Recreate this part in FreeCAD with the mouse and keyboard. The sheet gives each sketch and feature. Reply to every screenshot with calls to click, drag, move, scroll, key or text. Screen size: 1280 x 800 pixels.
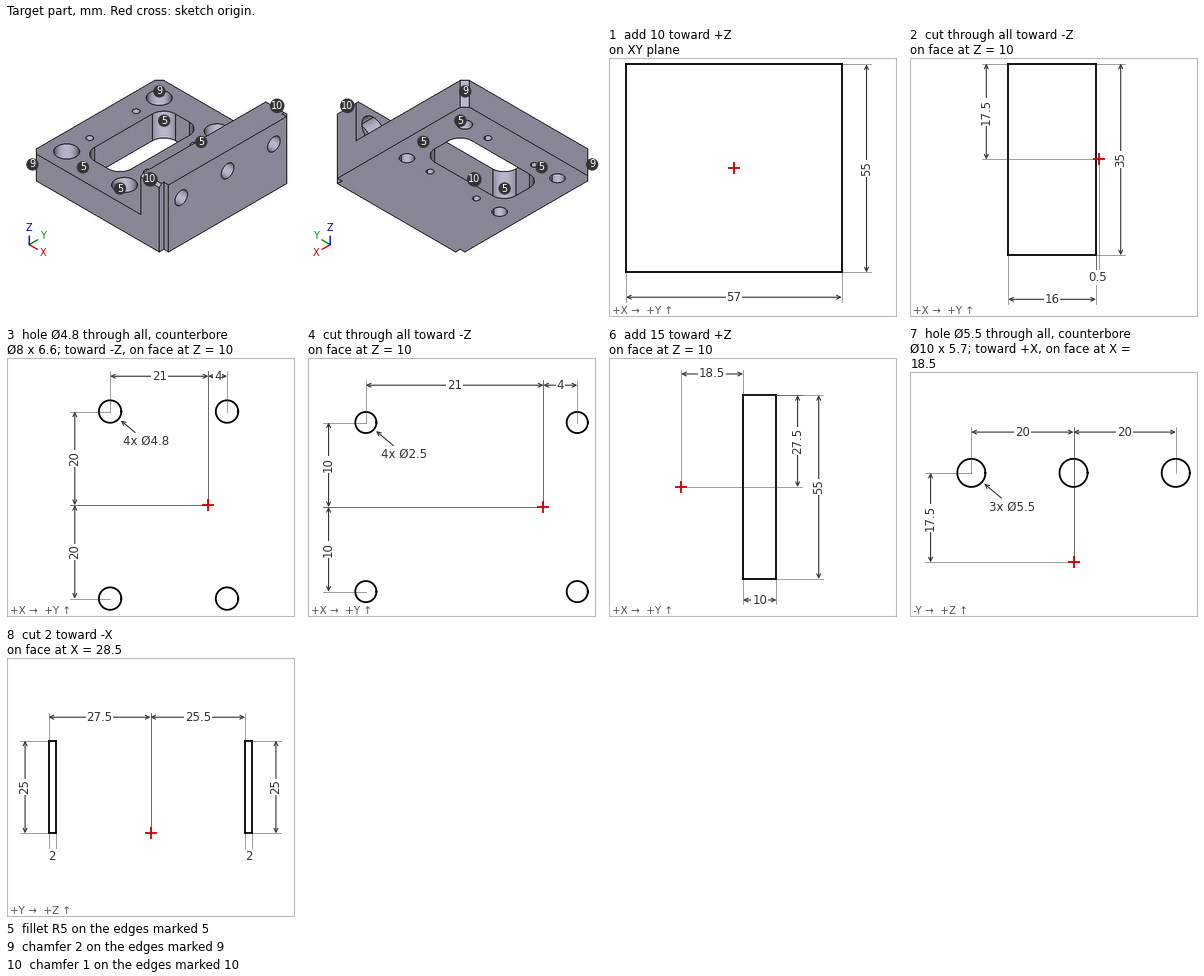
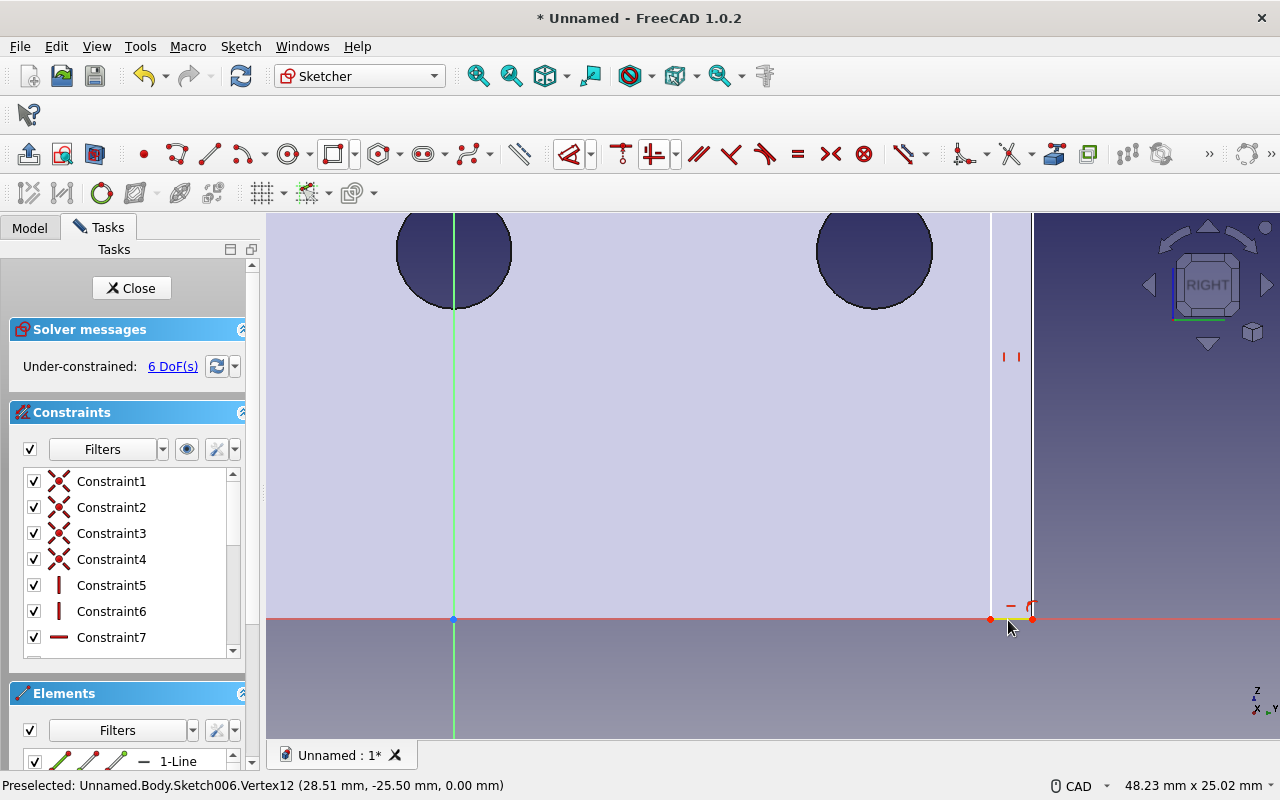
click(1008, 619)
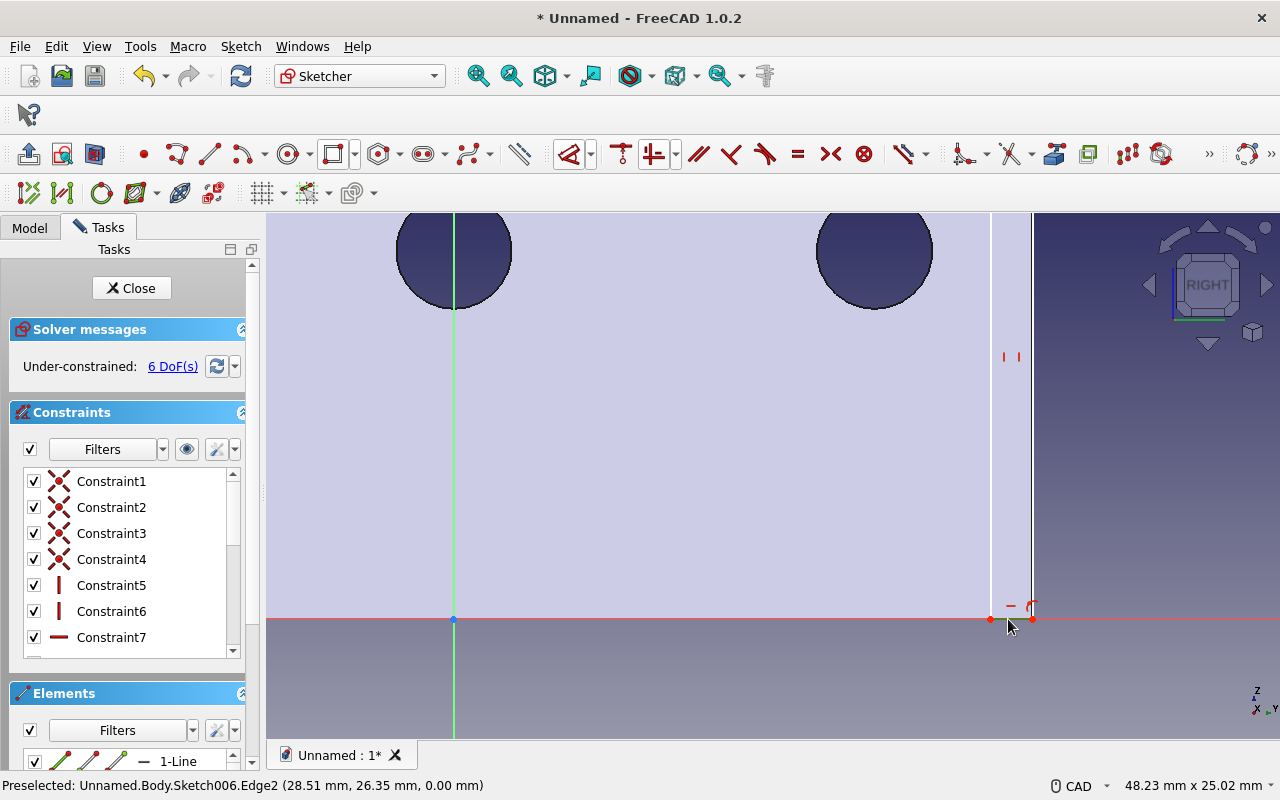
click(590, 154)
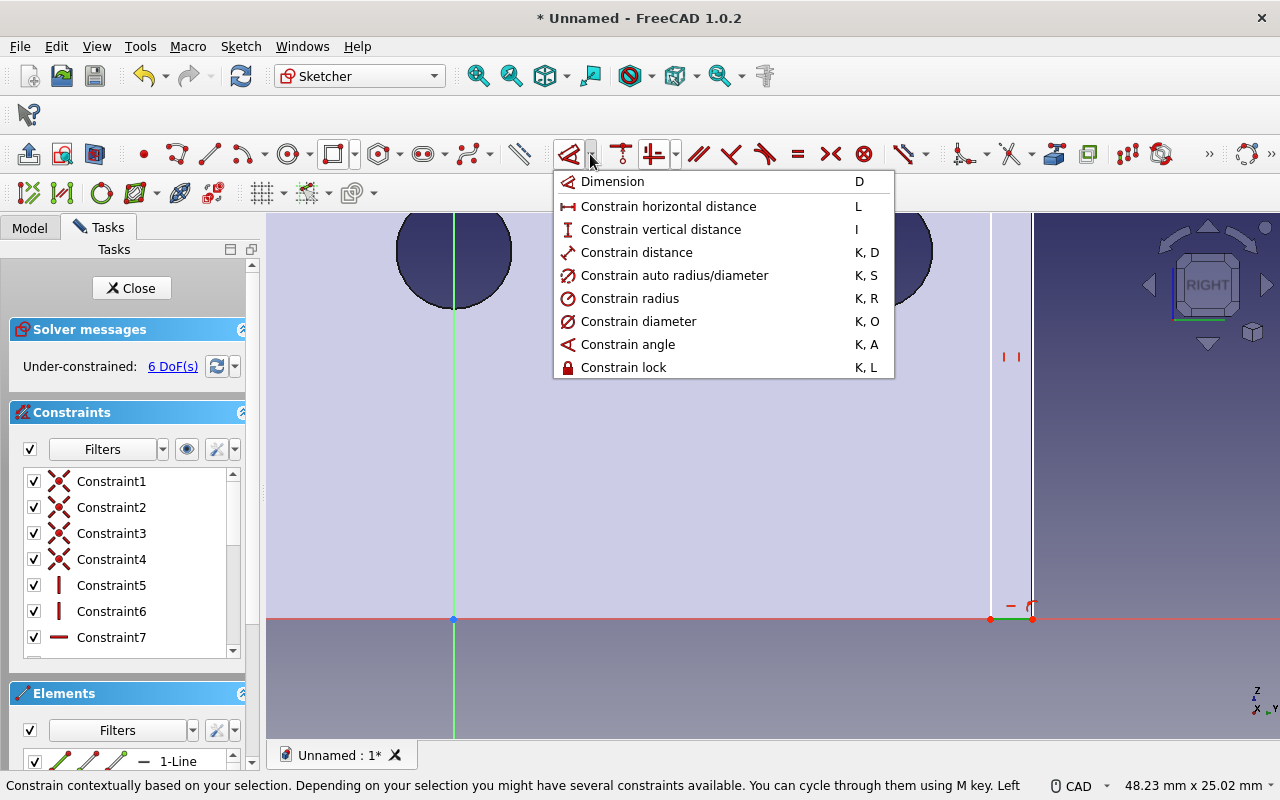
click(724, 206)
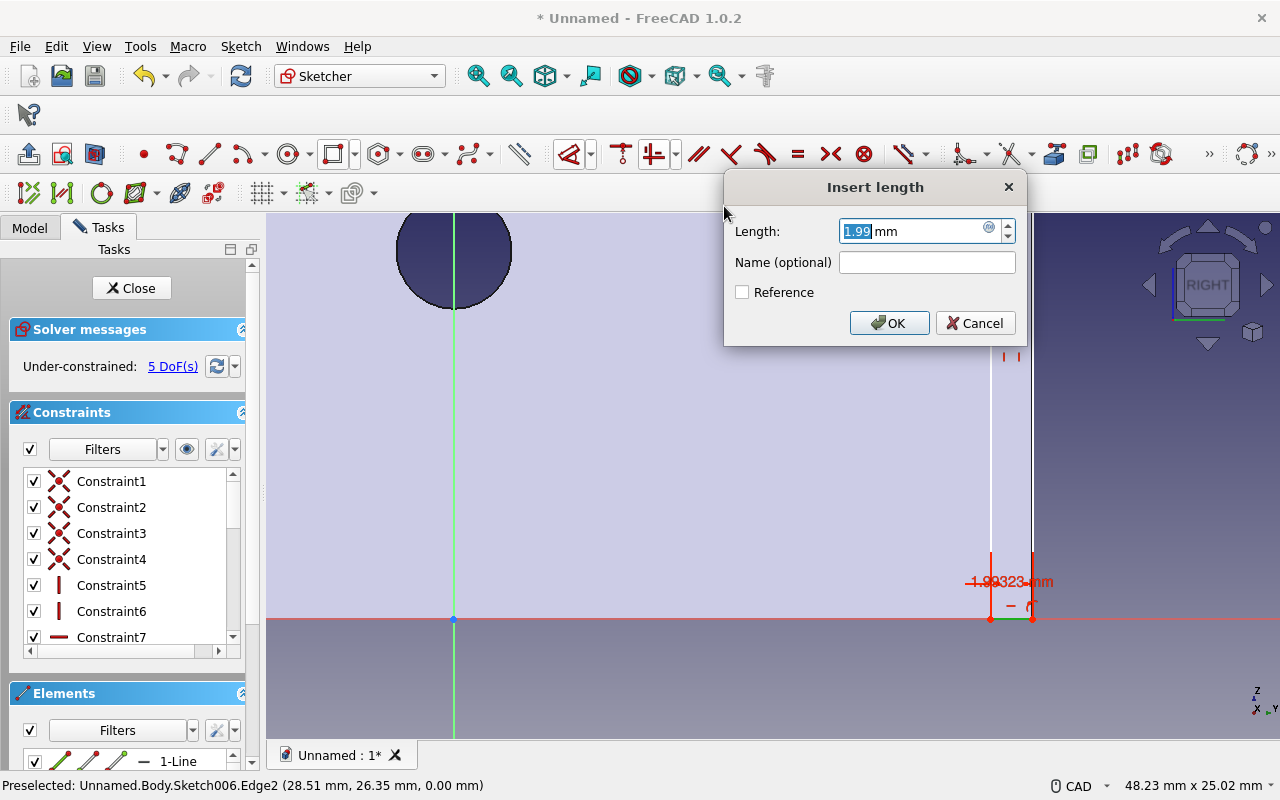
text(2)
key(Return)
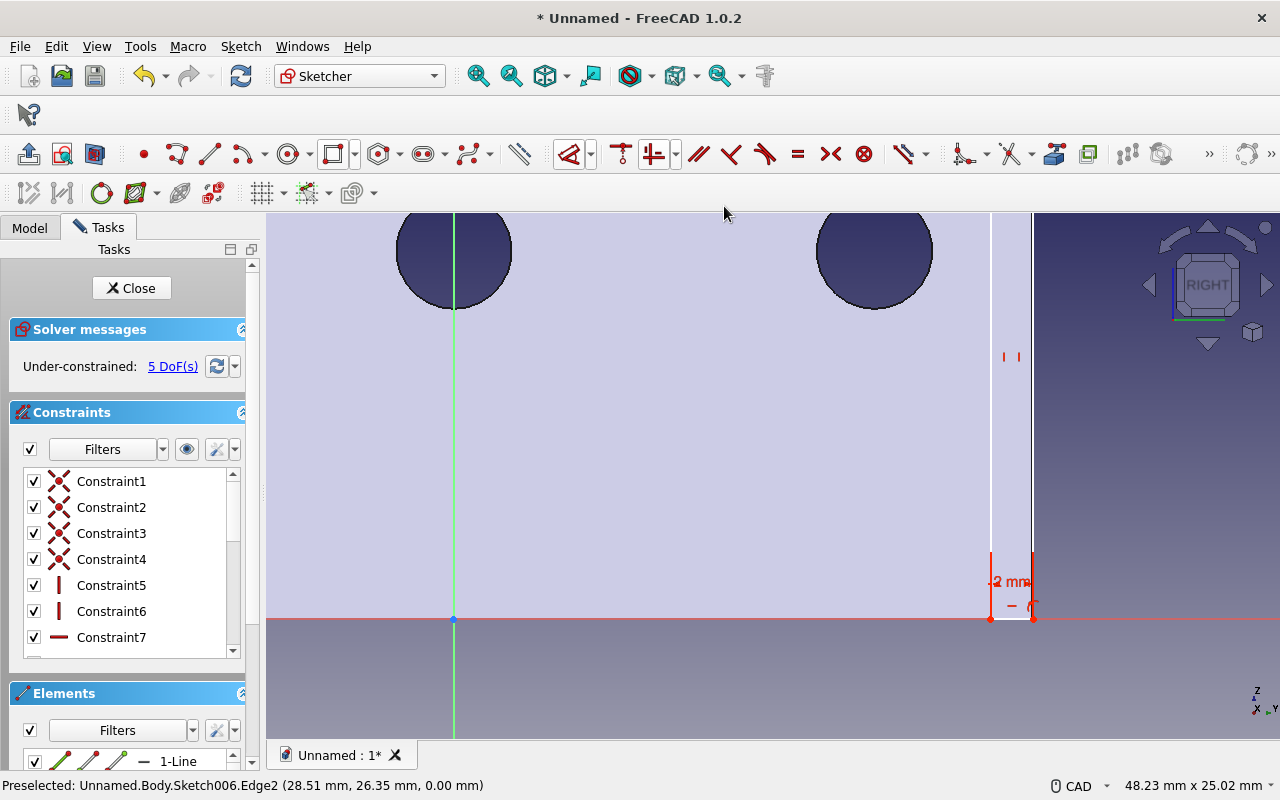
scroll(1009, 622, down, 3)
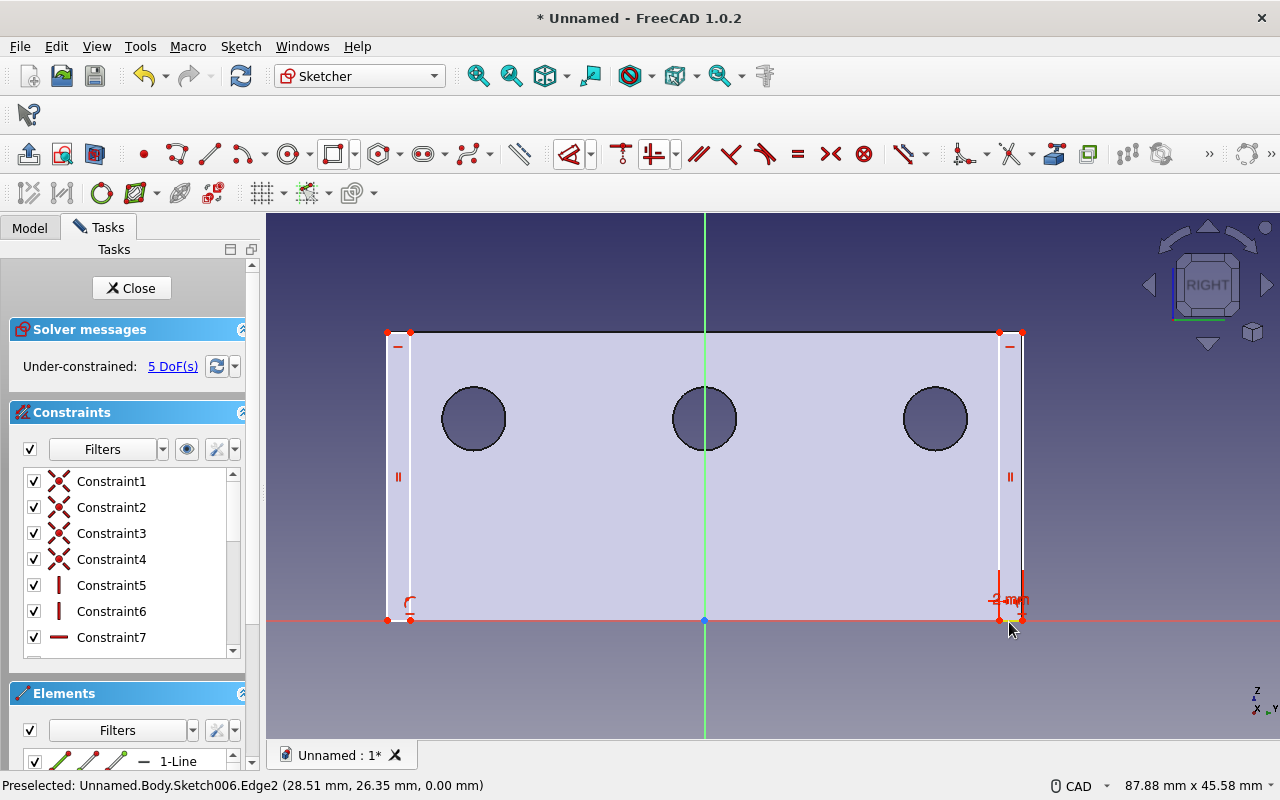
scroll(394, 621, up, 4)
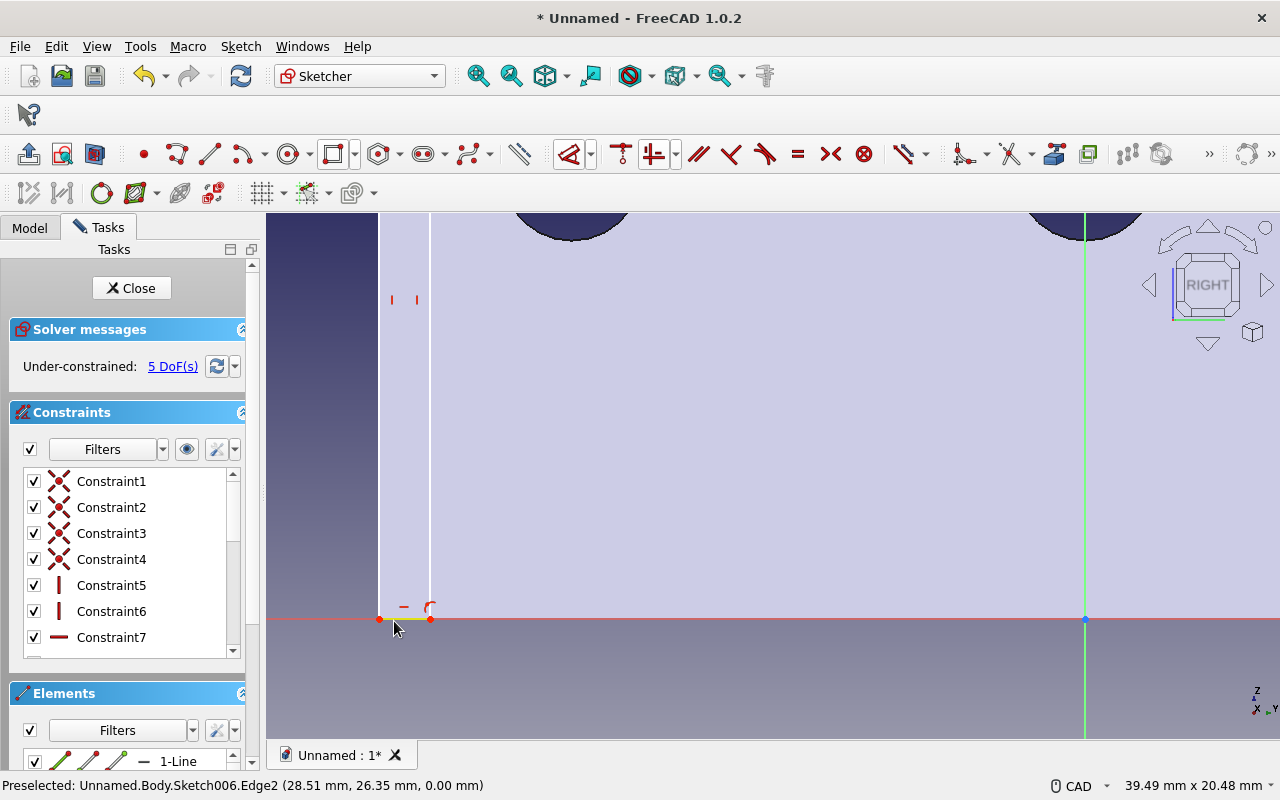
click(395, 619)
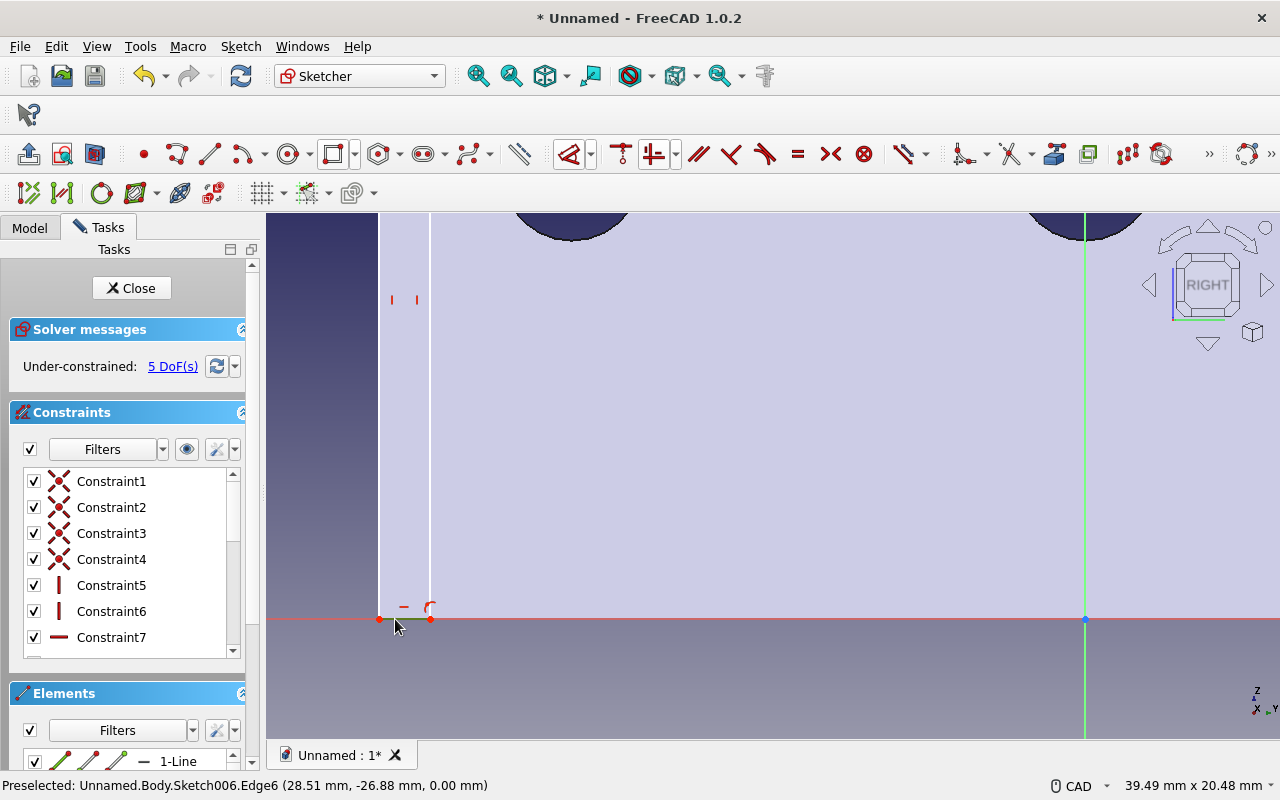
key(l)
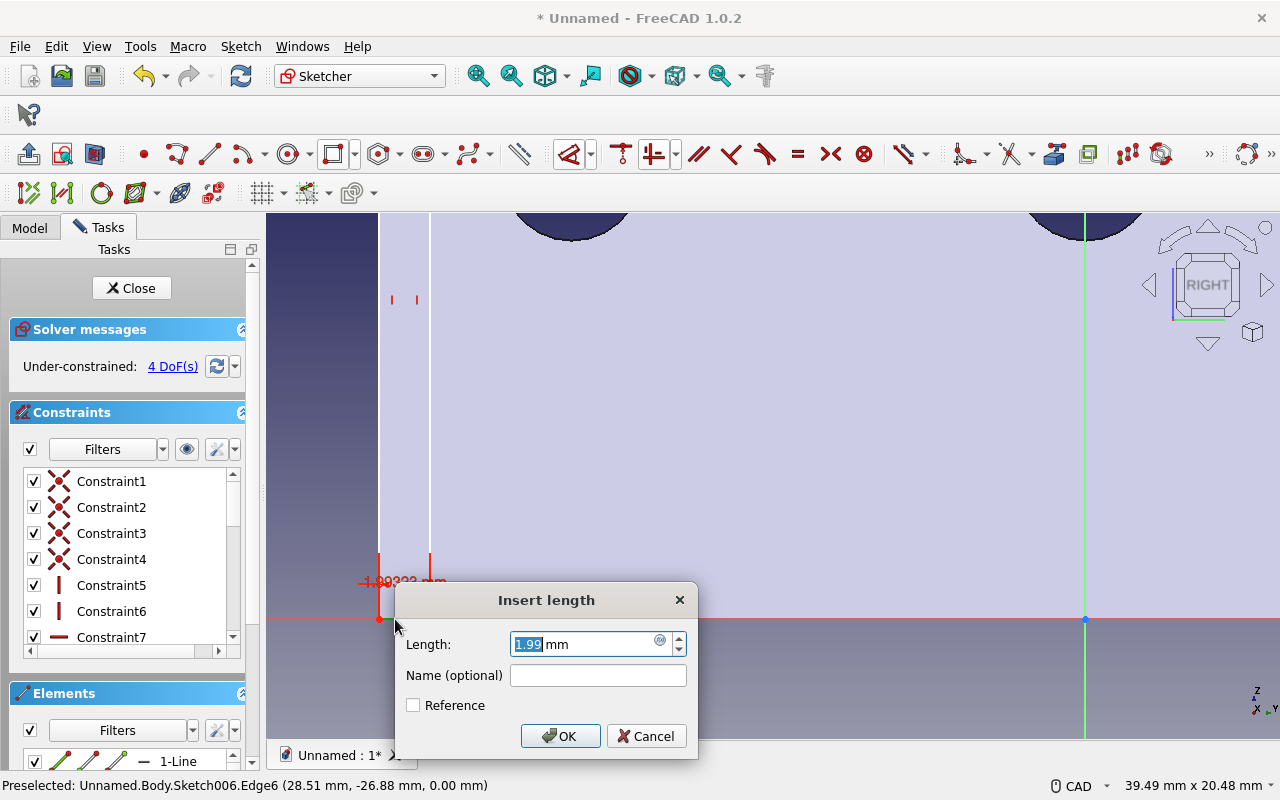
text(2)
key(Return)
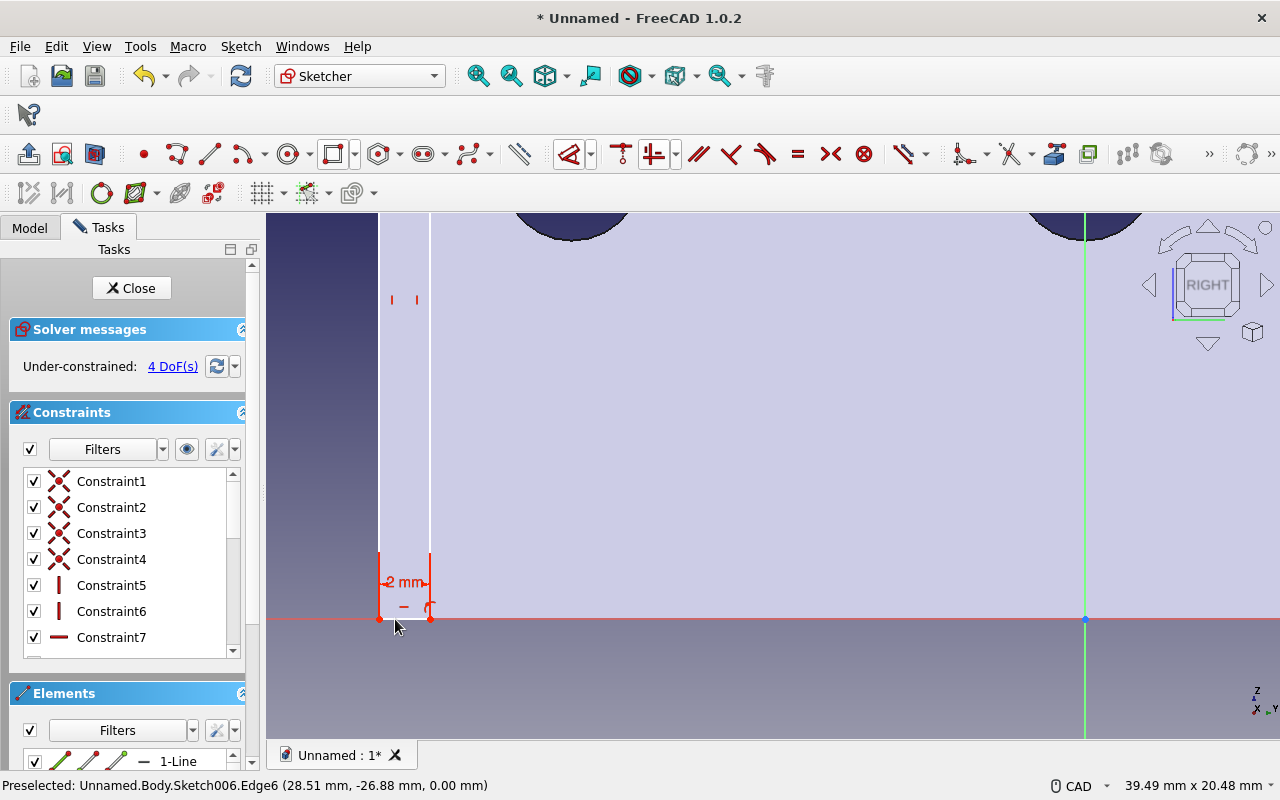
scroll(394, 621, down, 4)